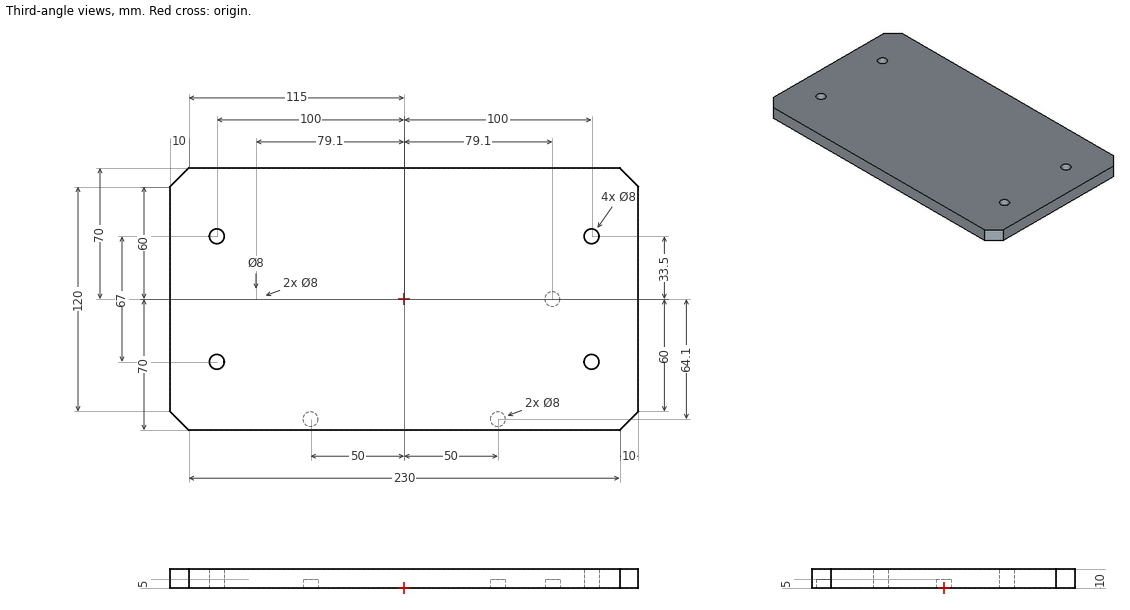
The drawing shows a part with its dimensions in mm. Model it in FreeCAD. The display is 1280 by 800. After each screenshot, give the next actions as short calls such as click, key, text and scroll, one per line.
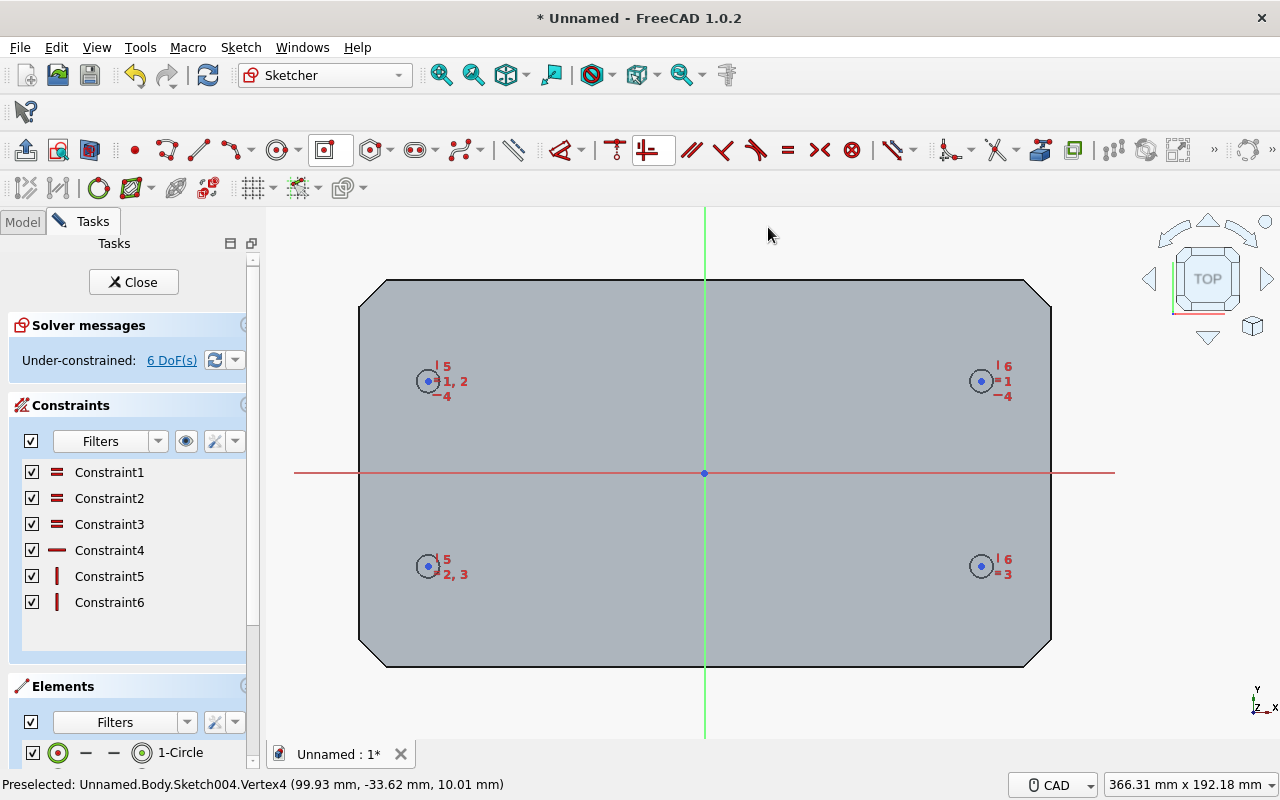
click(428, 566)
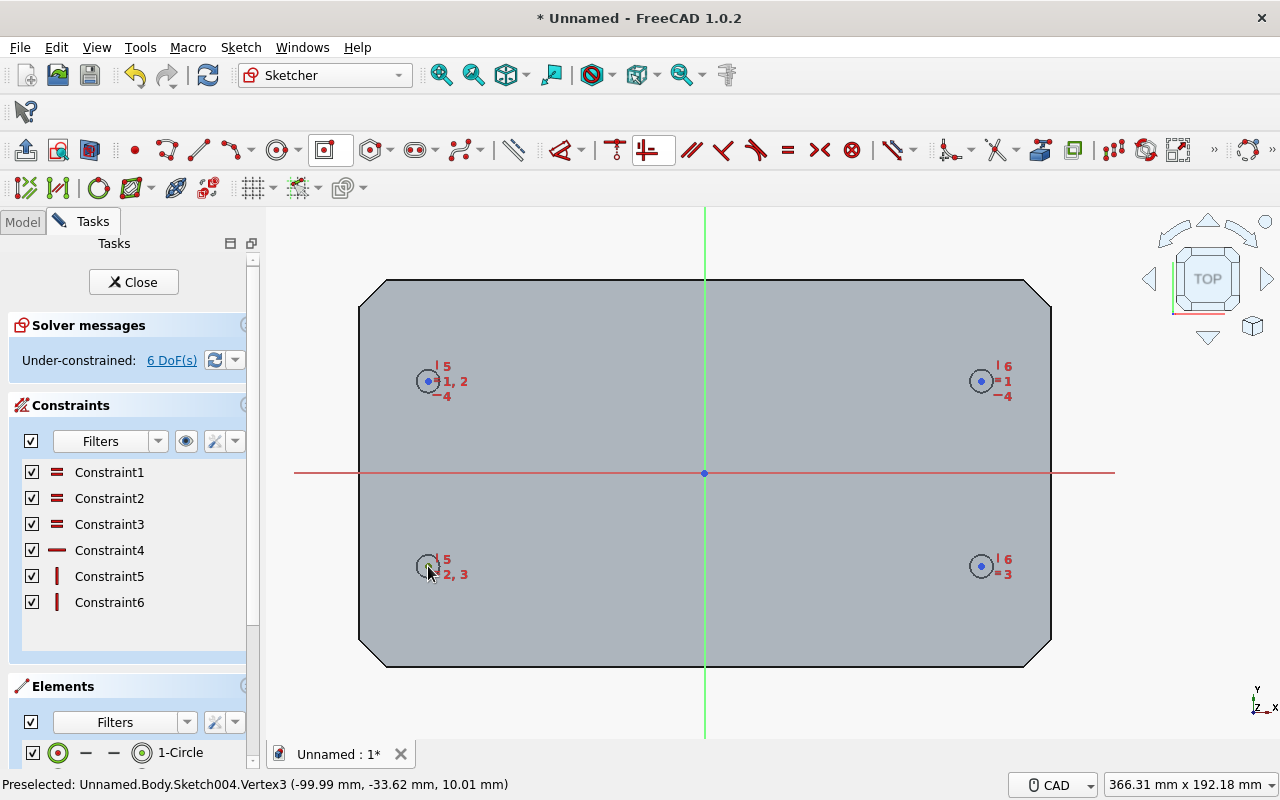
click(981, 566)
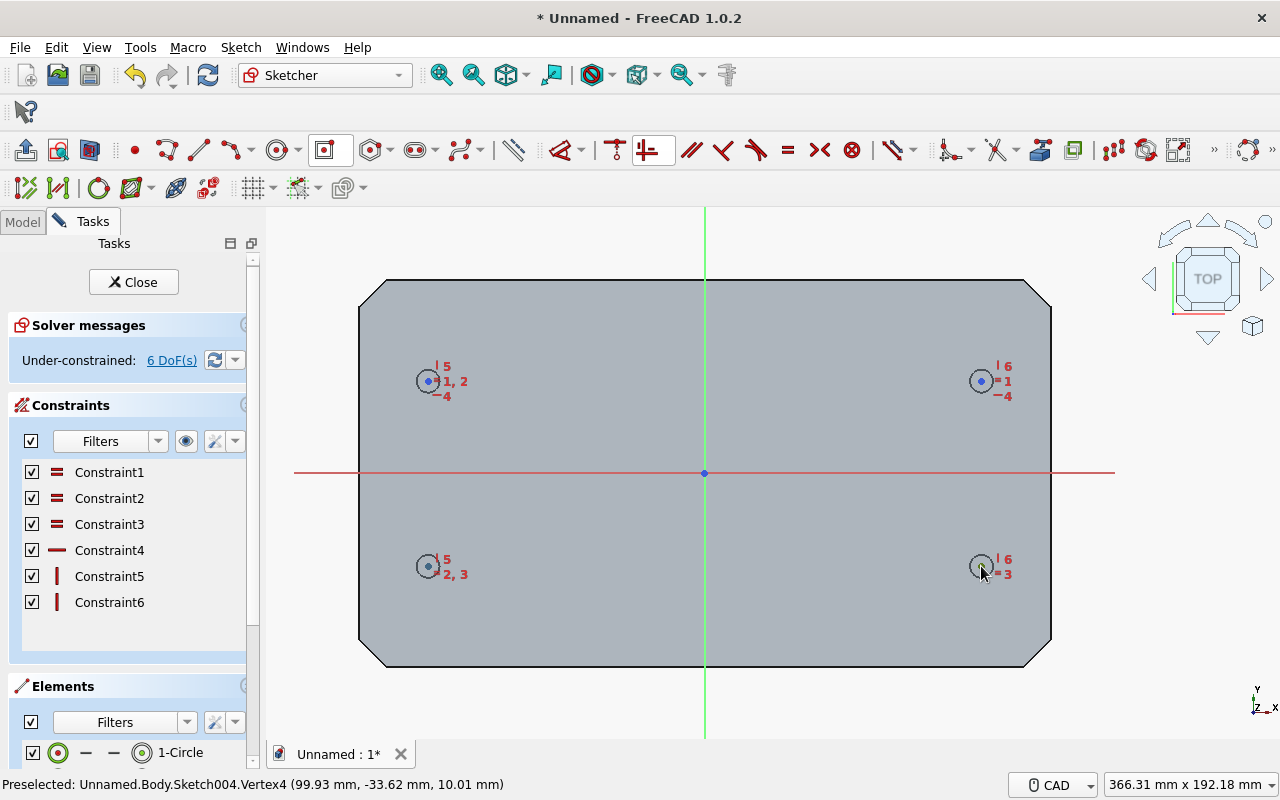
click(670, 150)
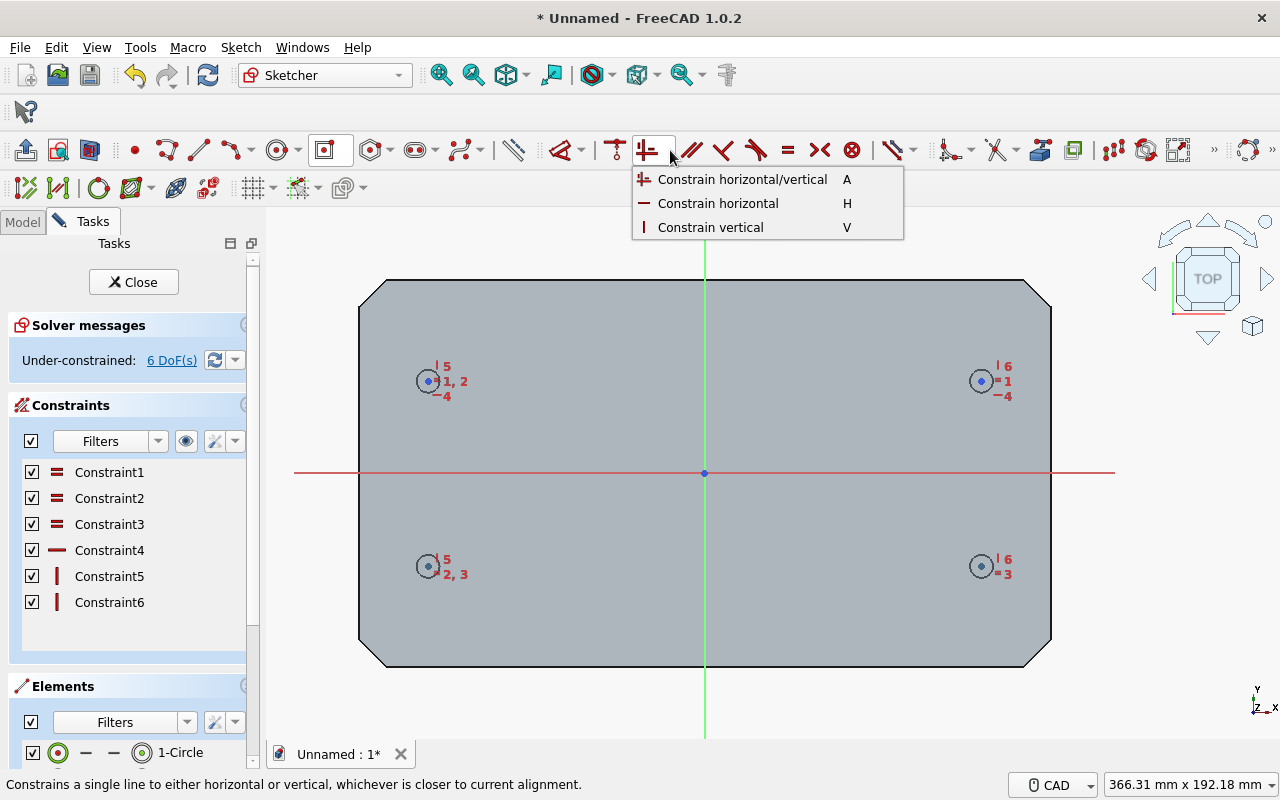
click(768, 203)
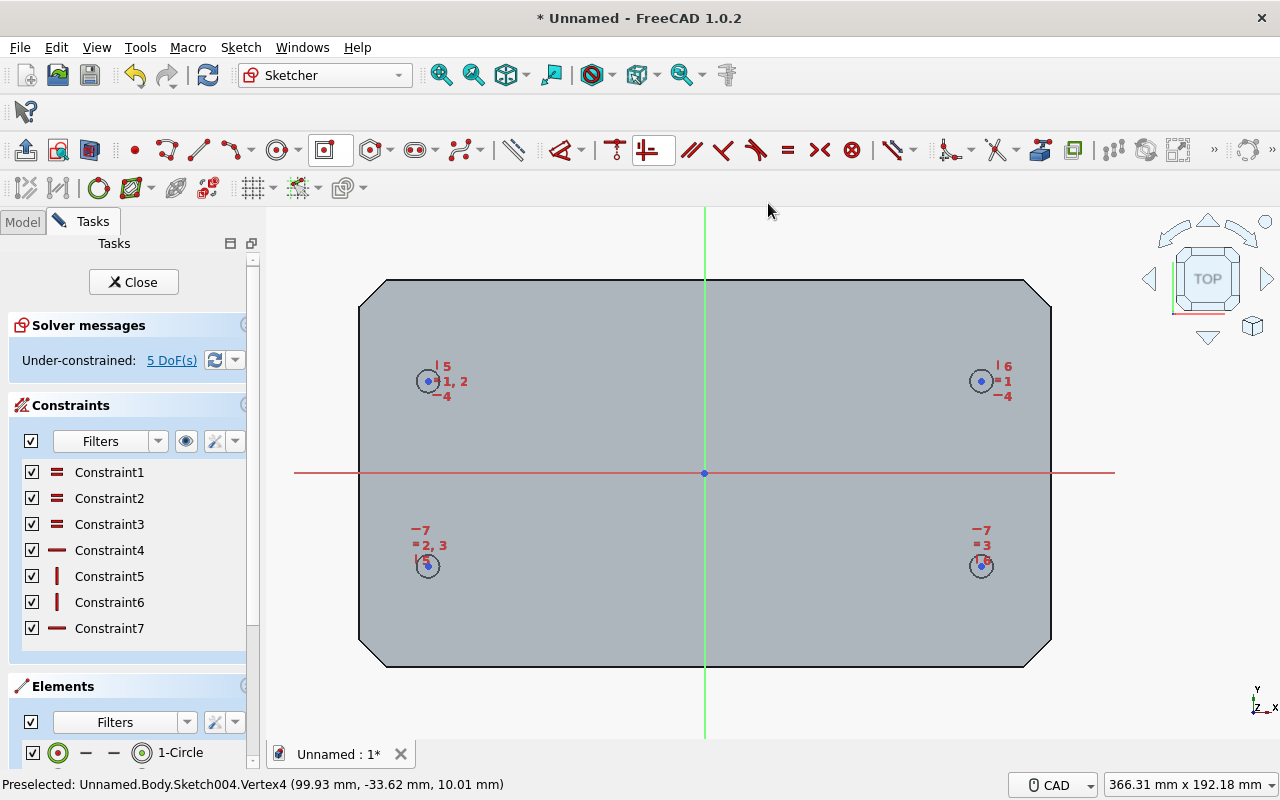
click(560, 150)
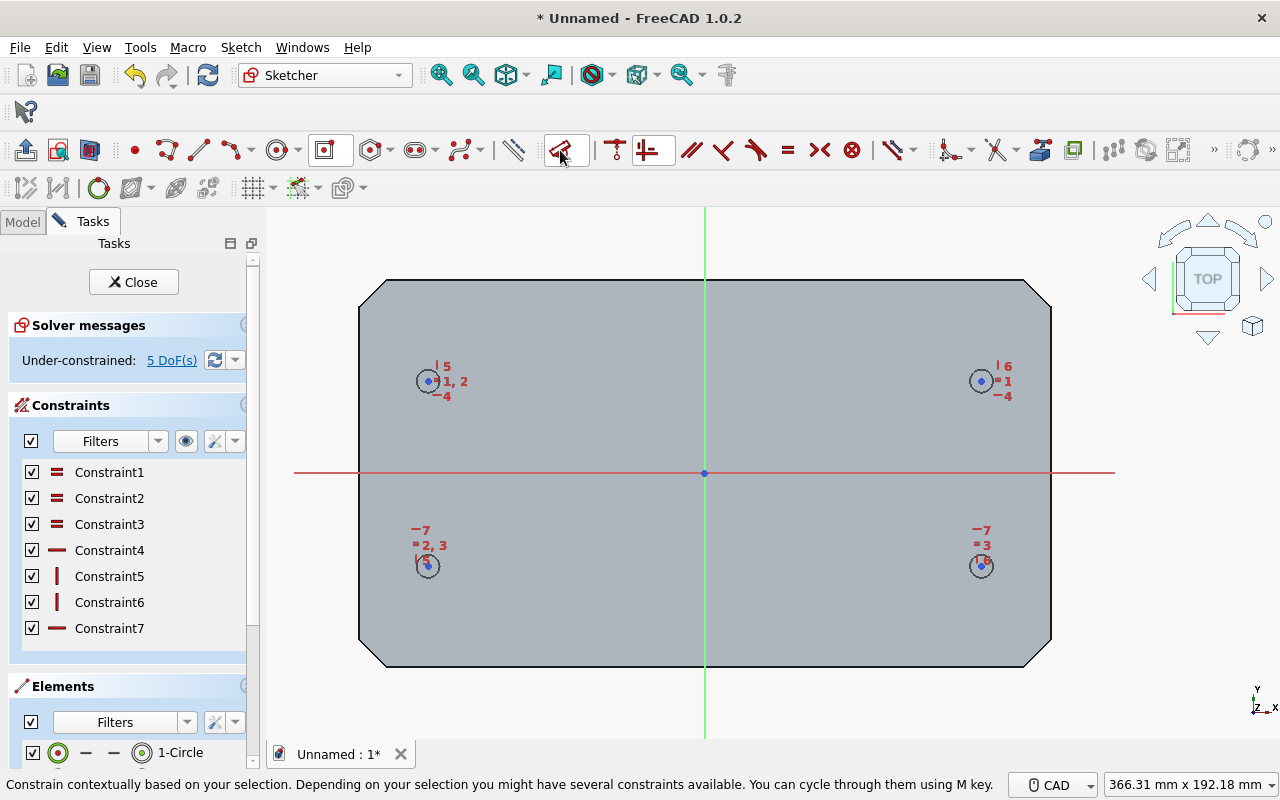
scroll(990, 373, up, 3)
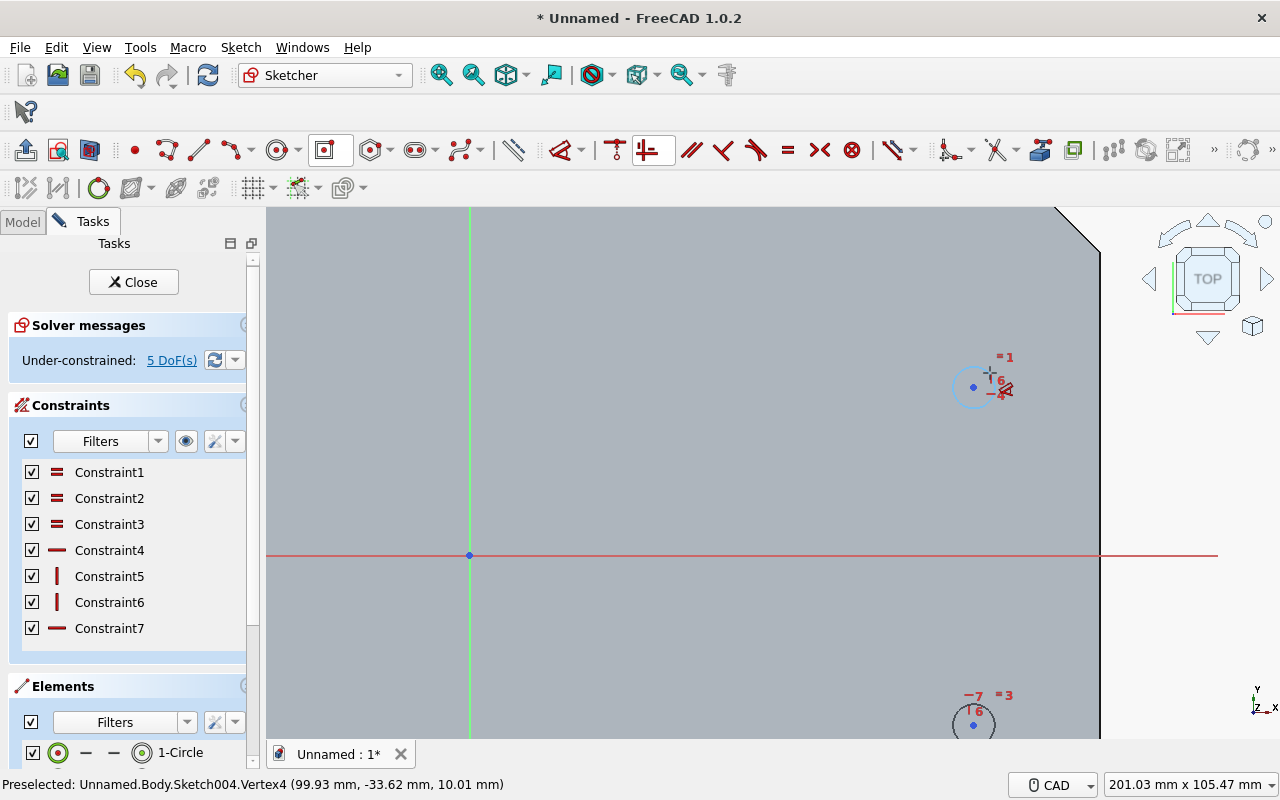
click(989, 373)
click(1012, 351)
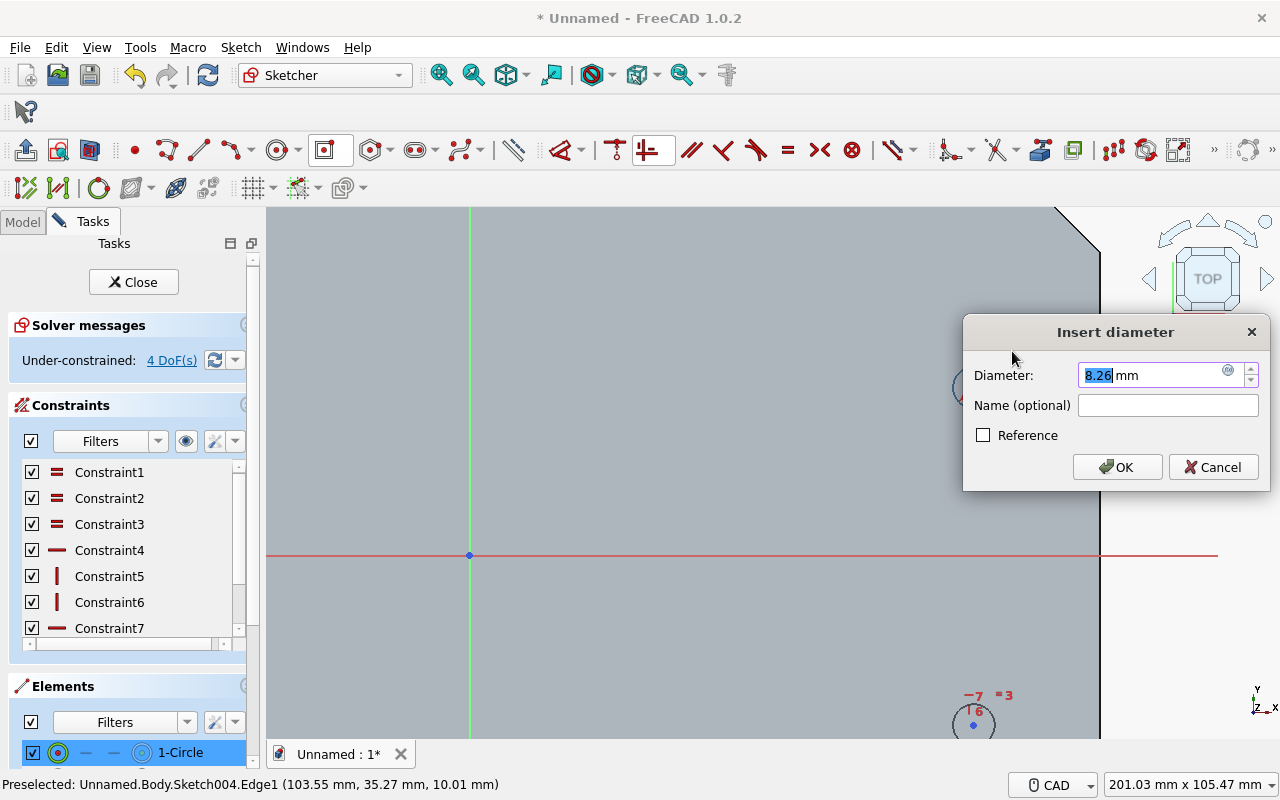
text(8)
key(Return)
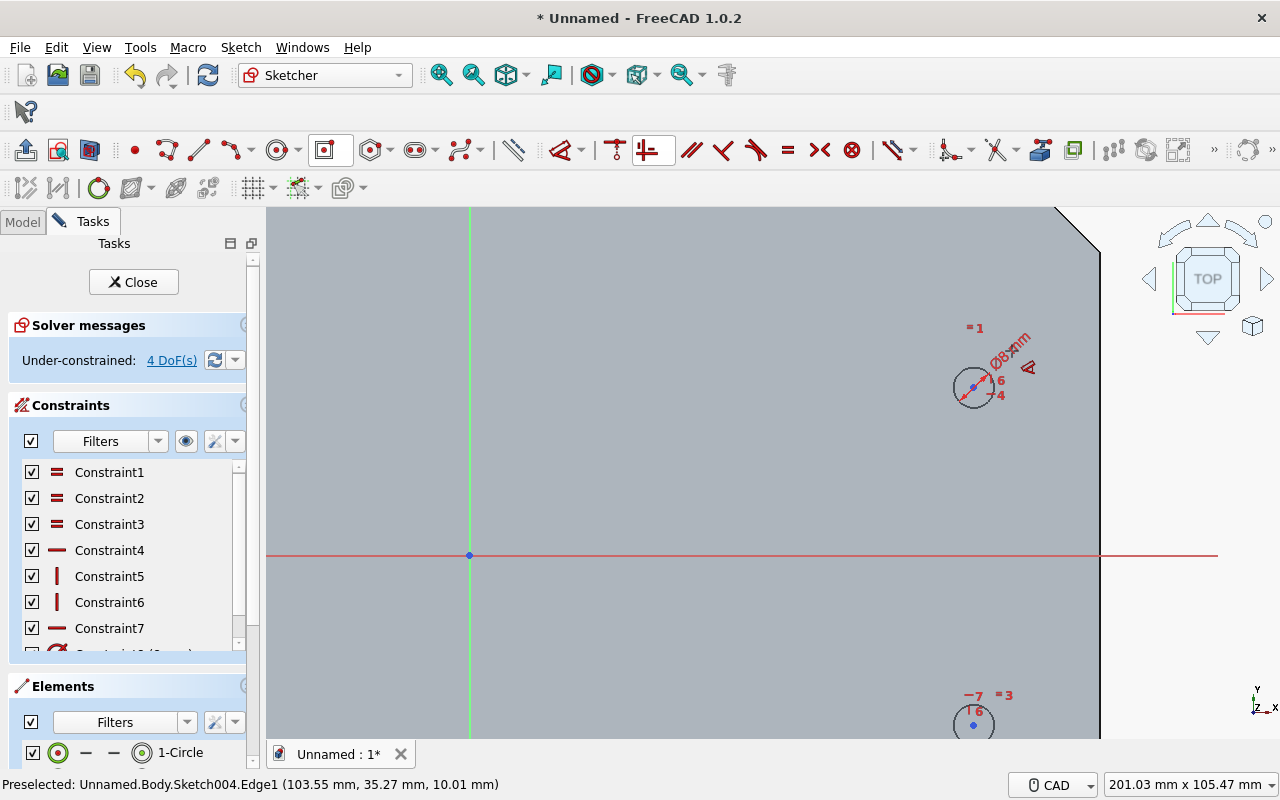
click(974, 388)
click(722, 354)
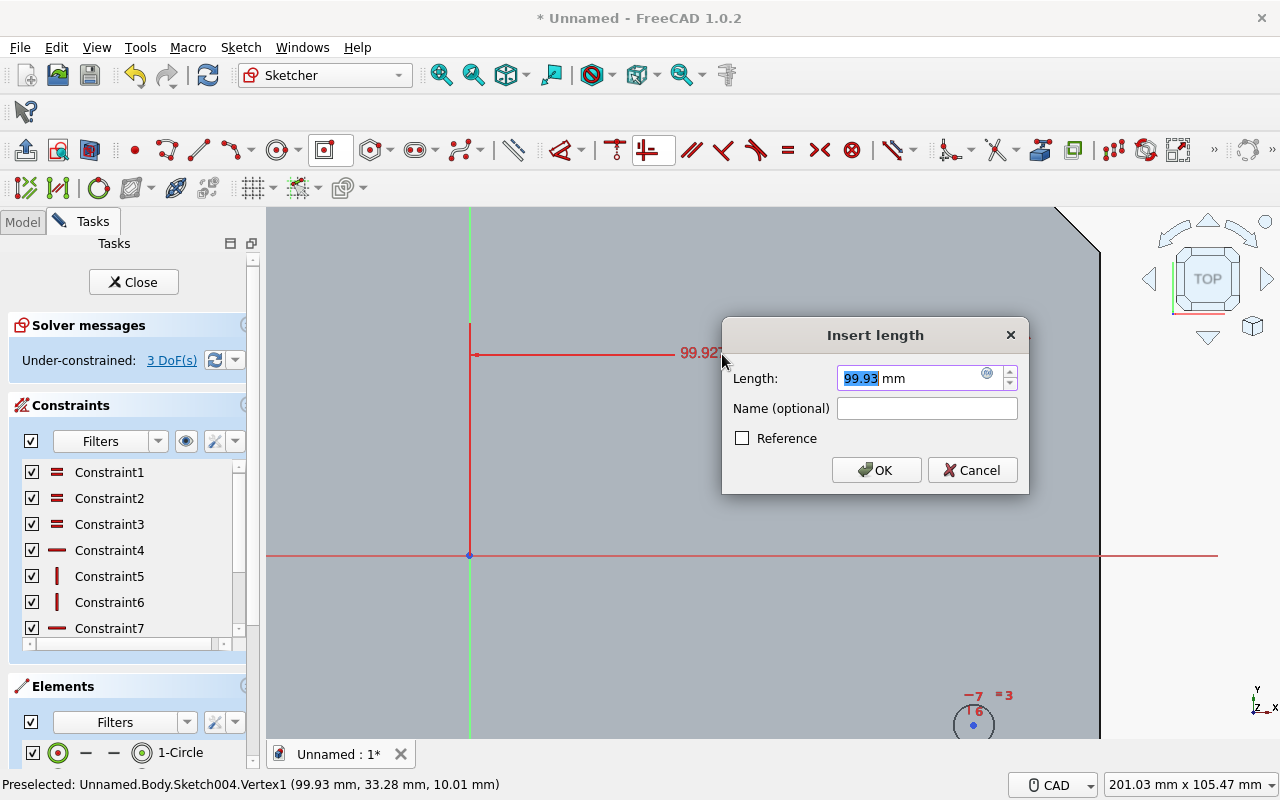
text(100)
key(Return)